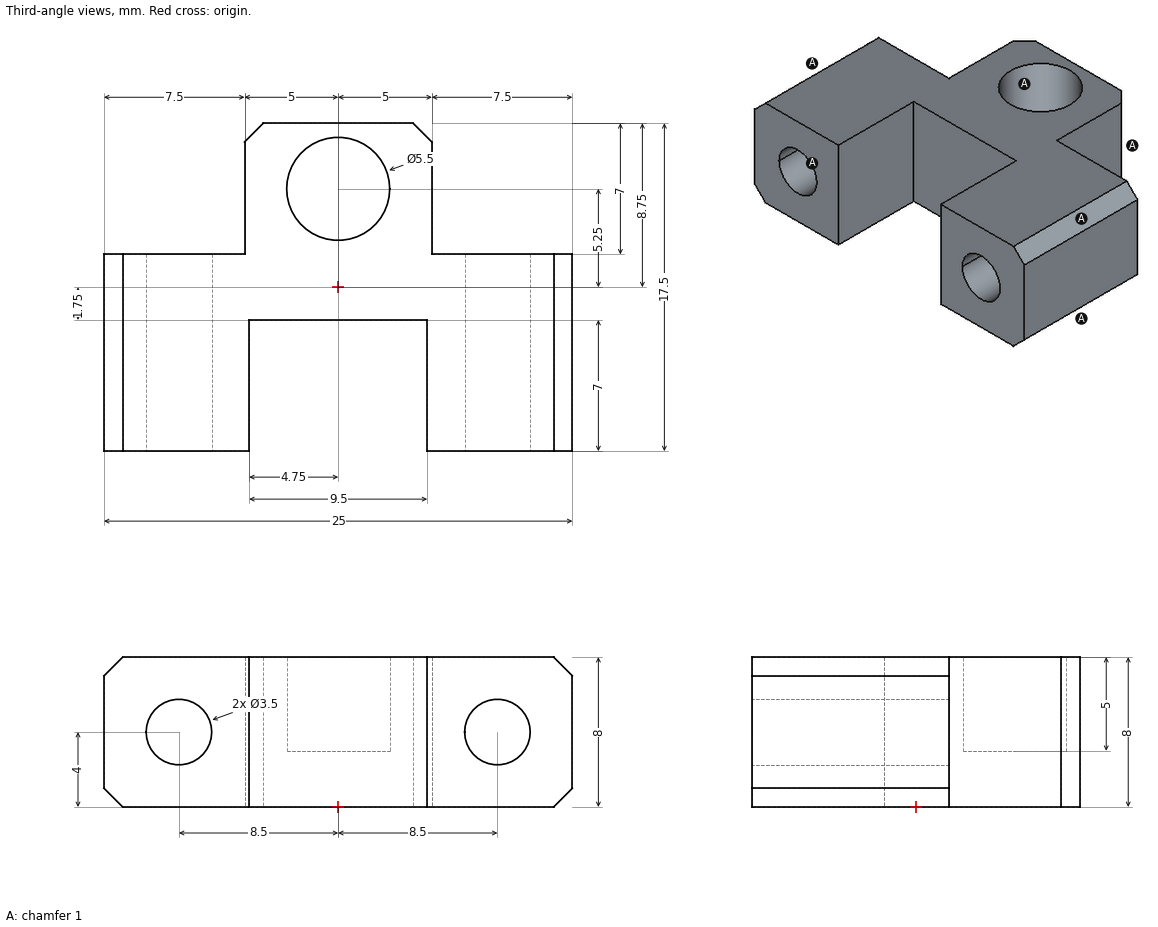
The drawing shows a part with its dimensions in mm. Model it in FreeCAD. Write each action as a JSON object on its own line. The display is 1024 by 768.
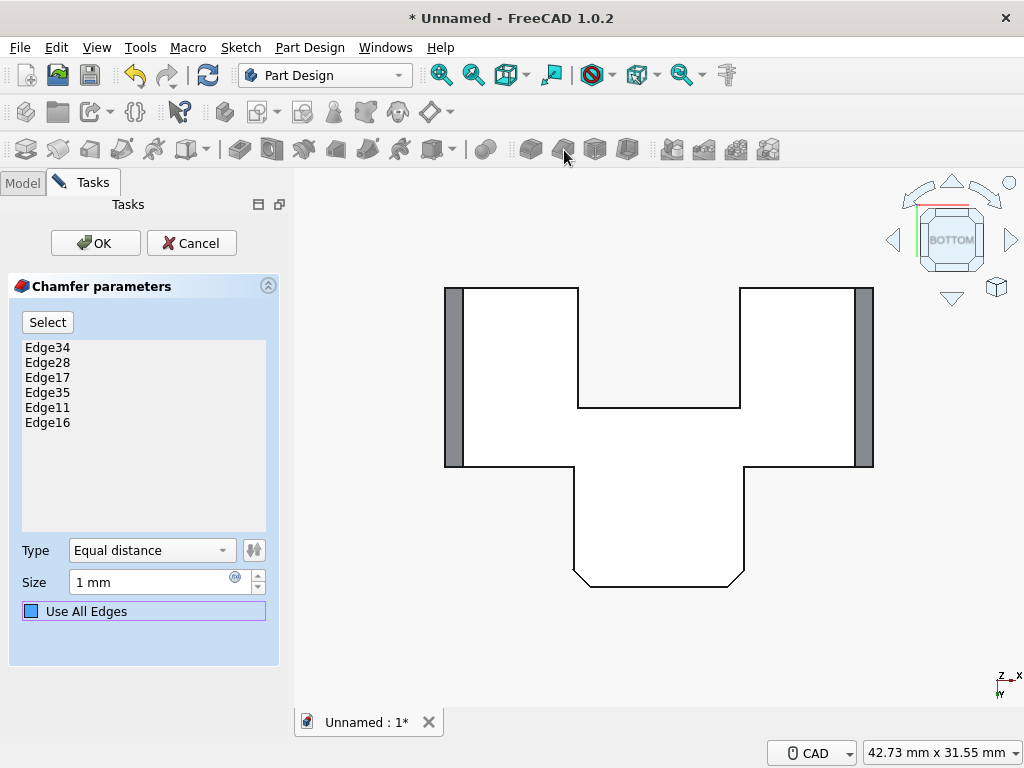
{"action": "left_click", "coordinate": [96, 243]}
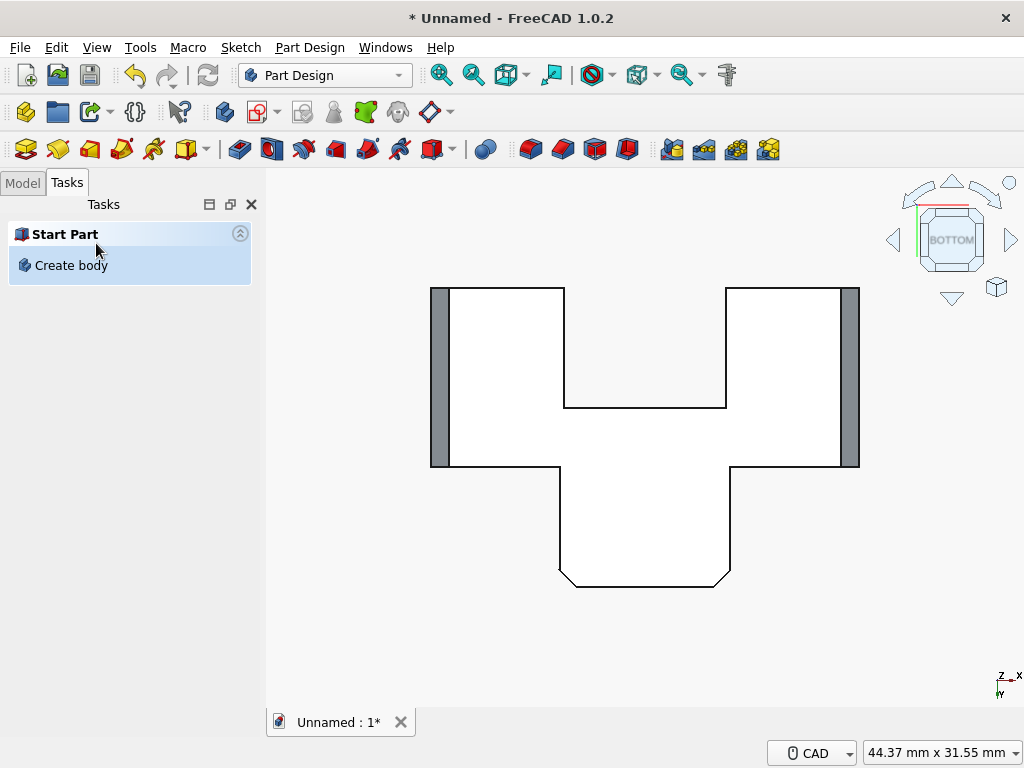
{"action": "key", "text": "0"}